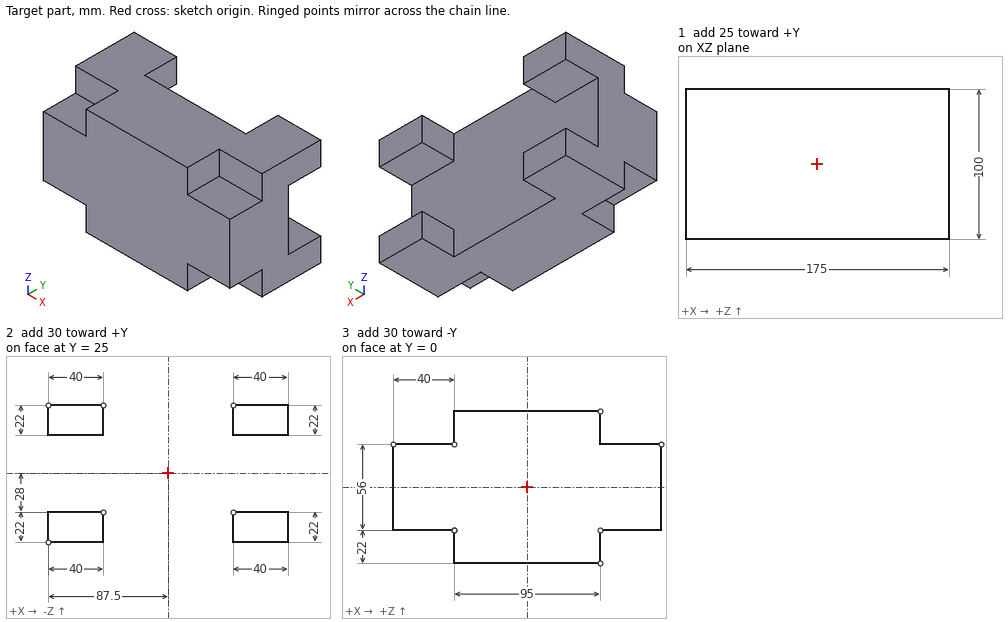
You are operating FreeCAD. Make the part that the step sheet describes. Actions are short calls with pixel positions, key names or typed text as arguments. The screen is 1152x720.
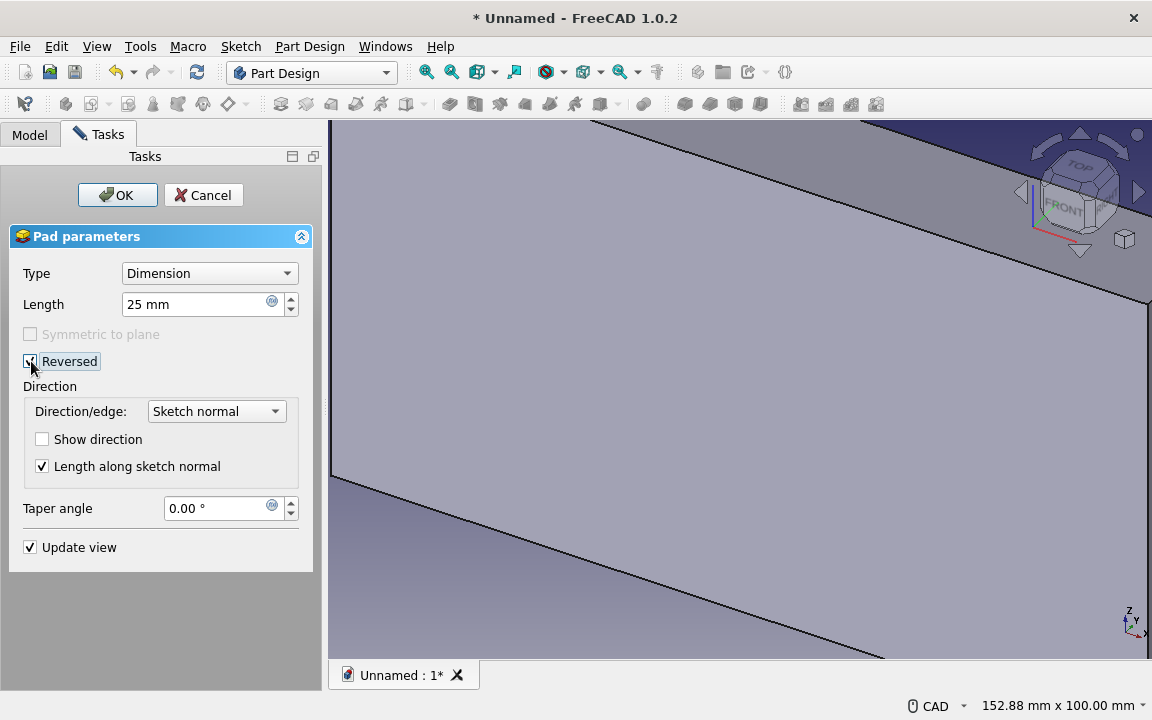
click(118, 195)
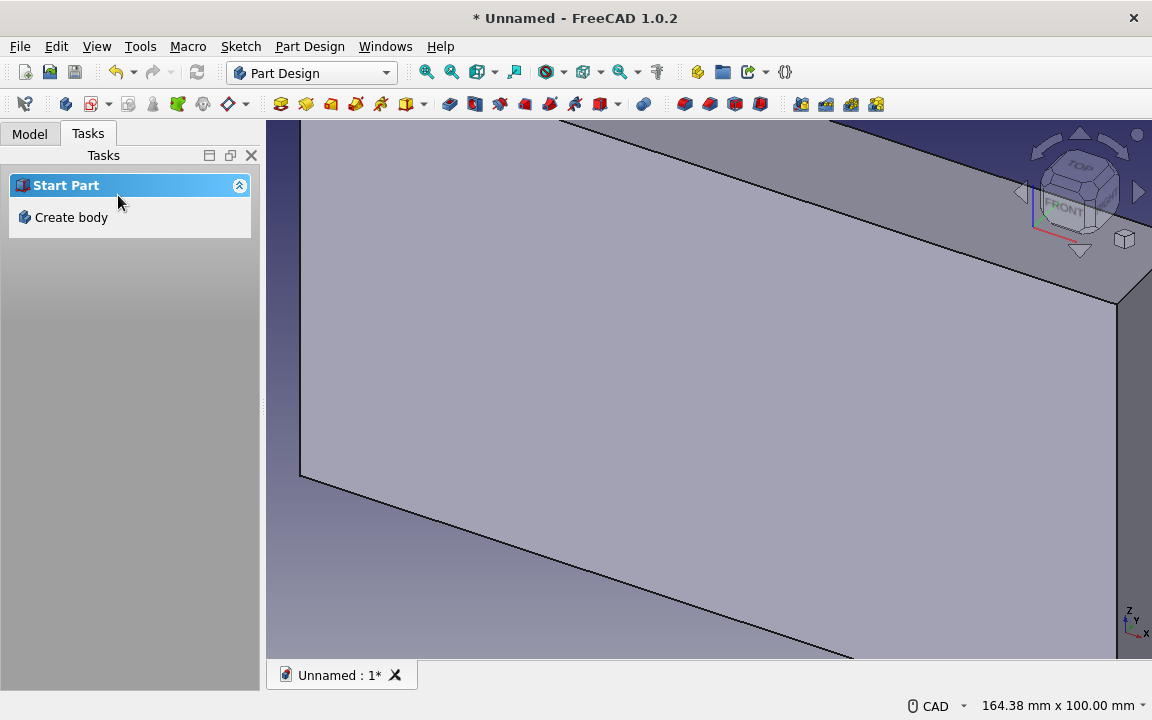
key(v)
key(f)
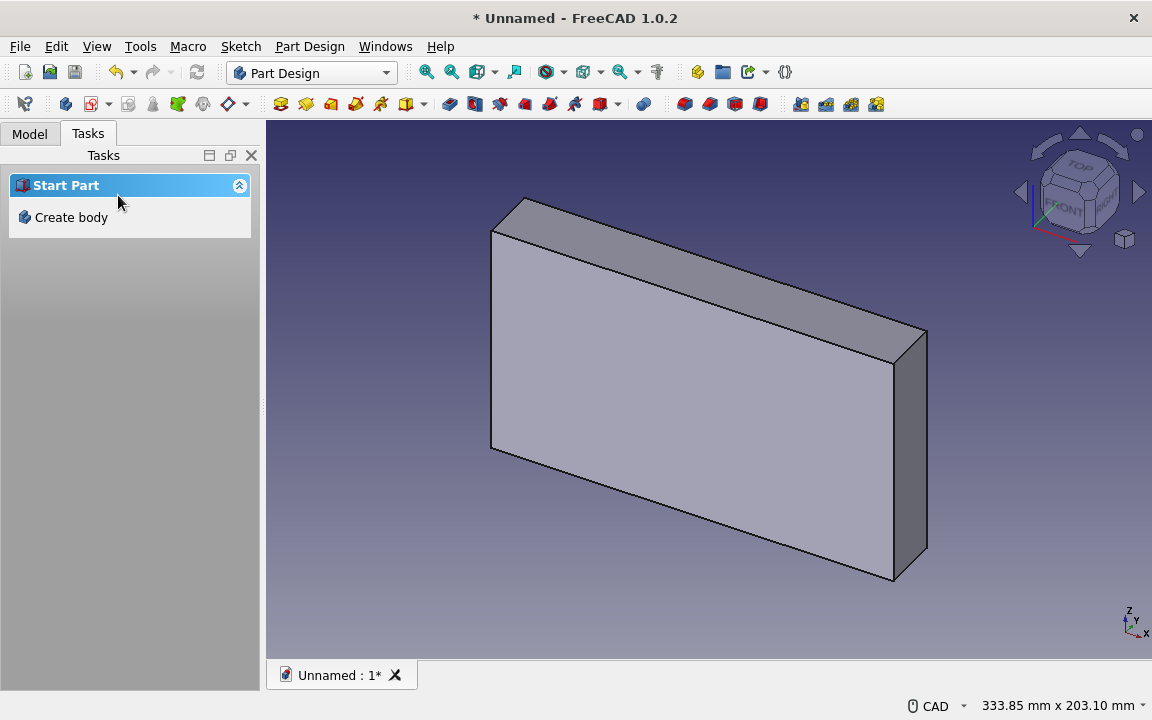
key(4)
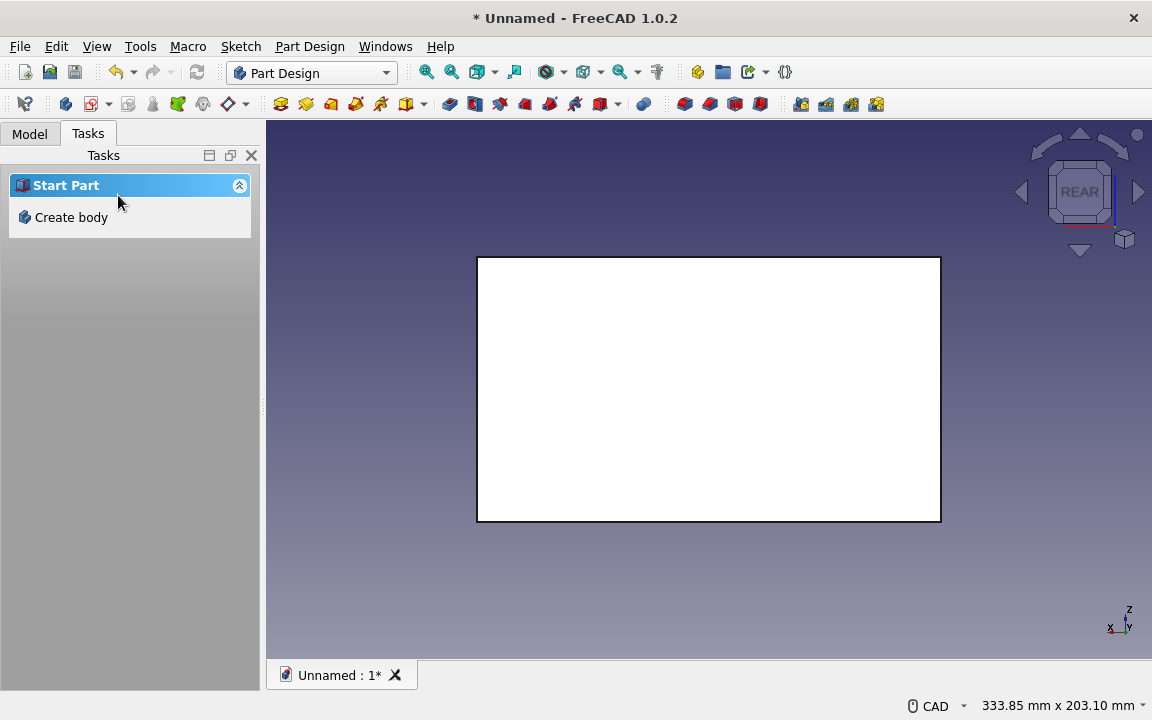
click(643, 389)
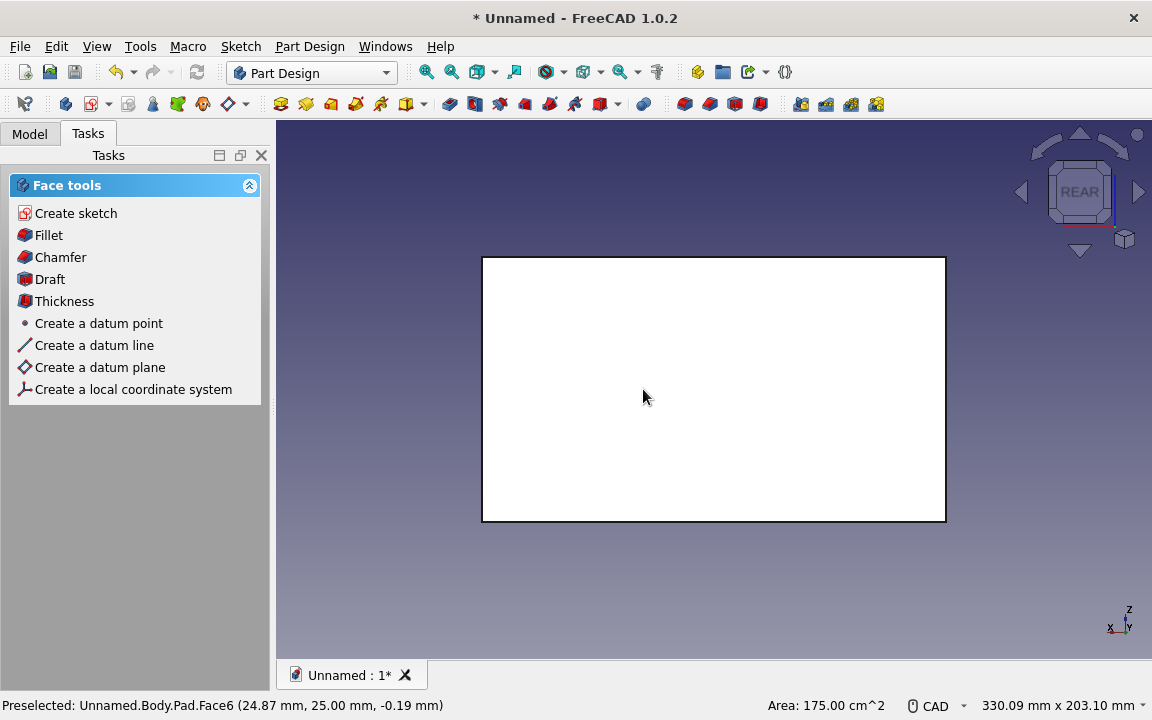
click(90, 104)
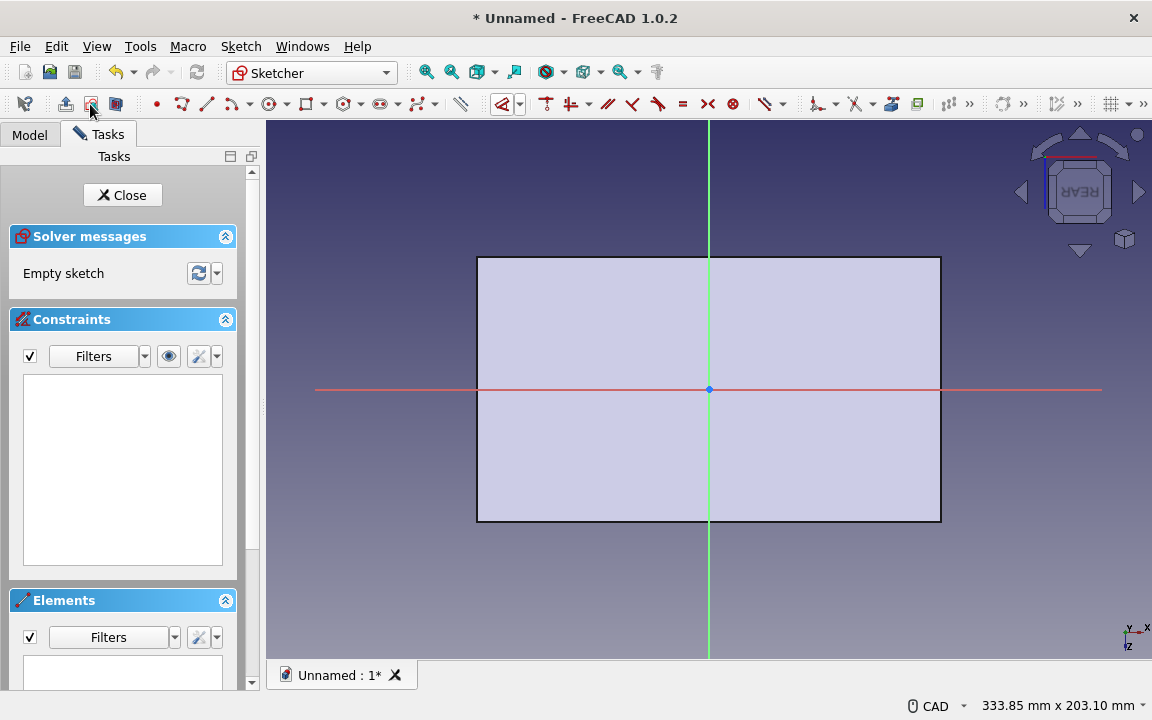
click(306, 104)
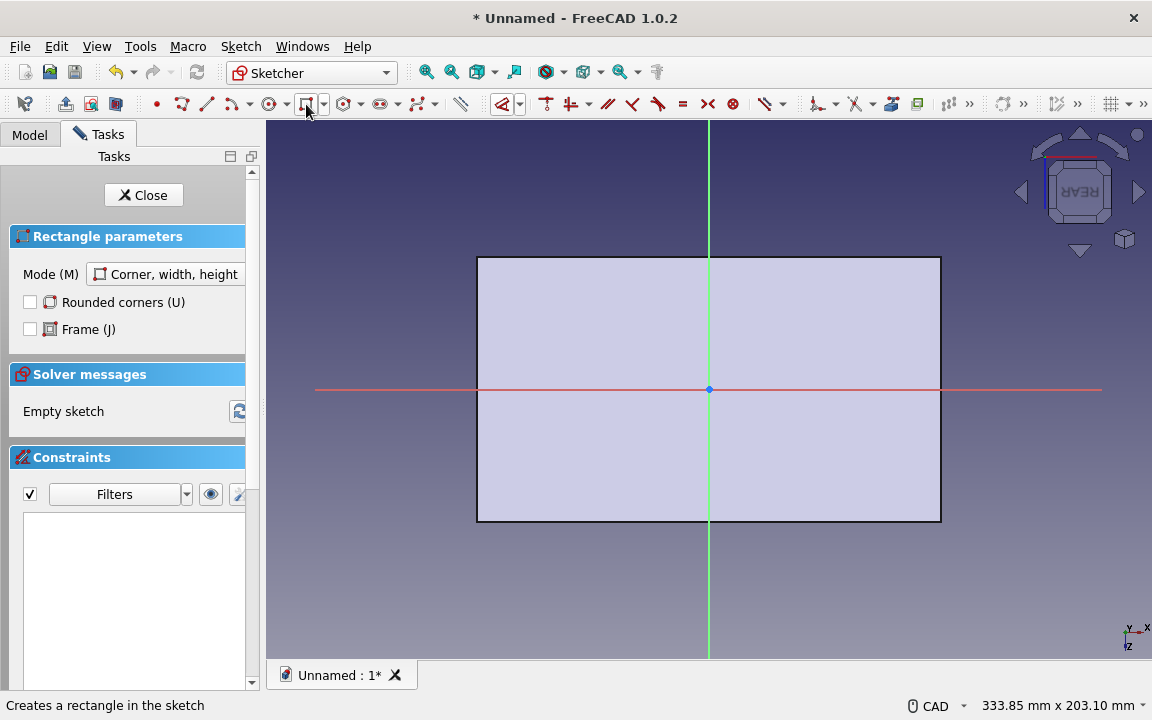
click(477, 464)
move(583, 522)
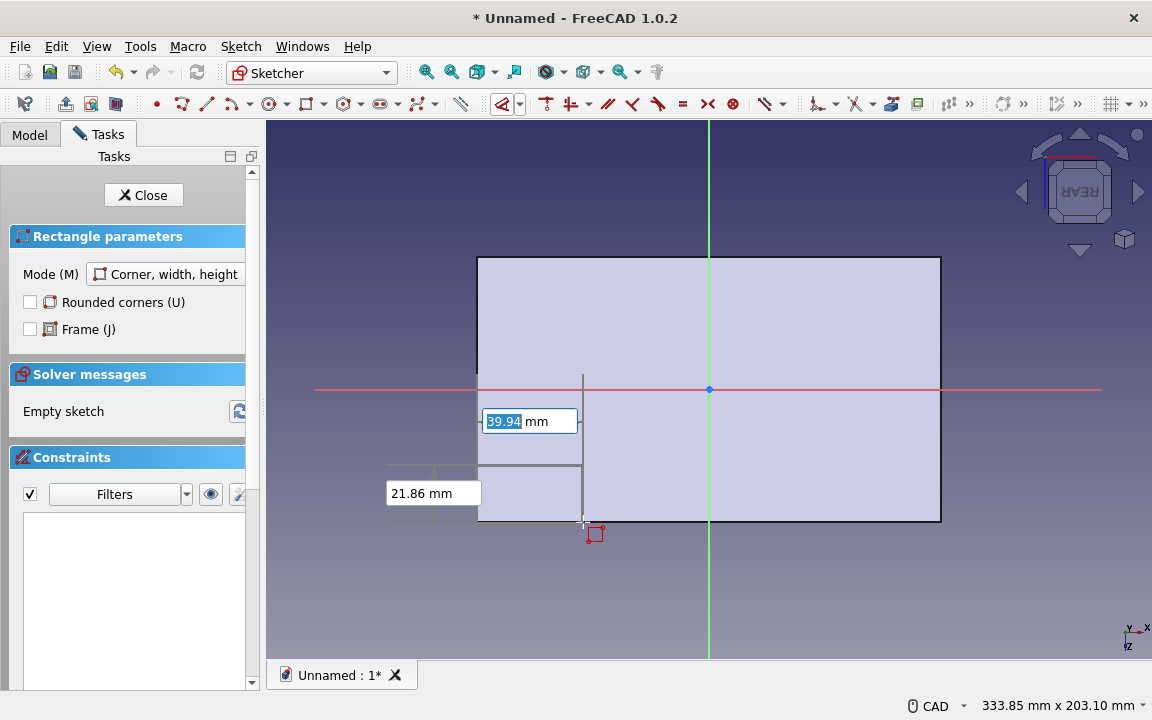
text(40)
key(Tab)
text(22)
key(Return)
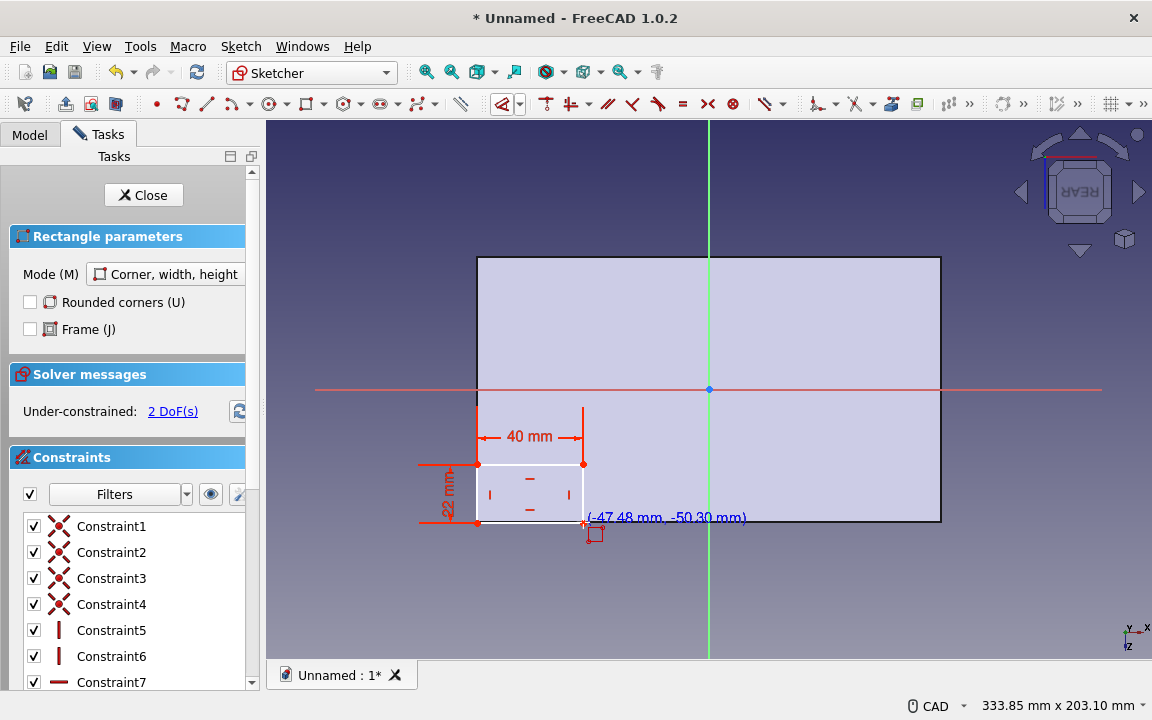
click(477, 257)
move(583, 315)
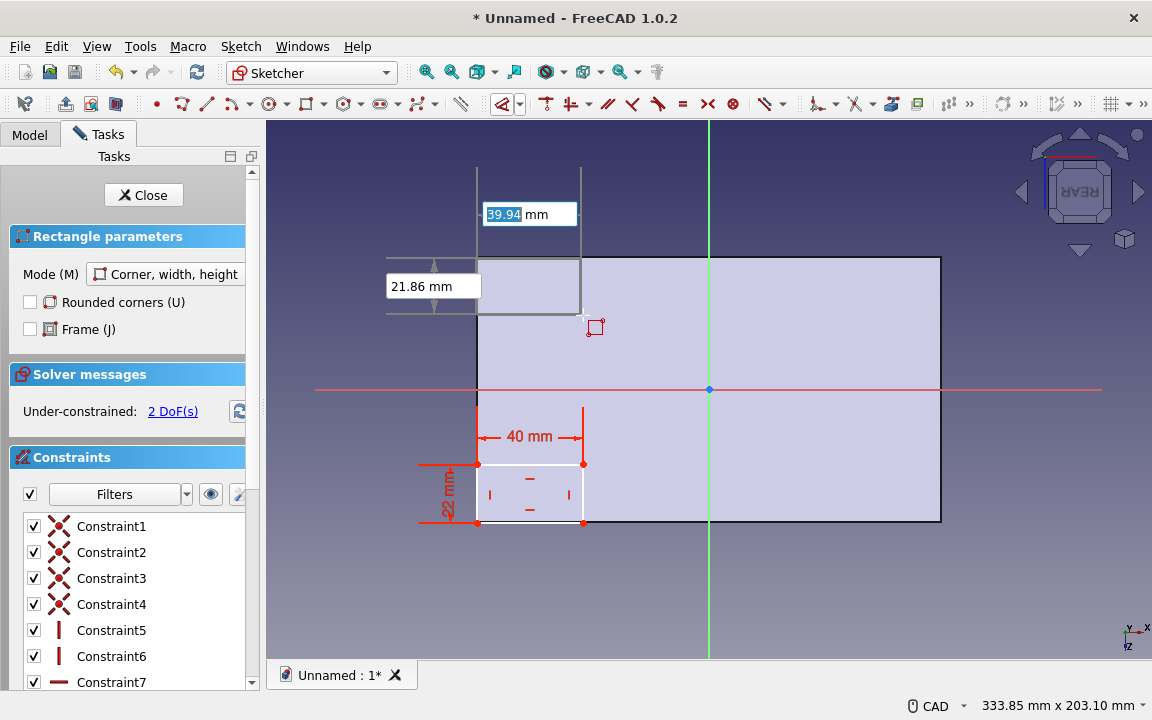
text(40)
key(Tab)
text(22)
key(Return)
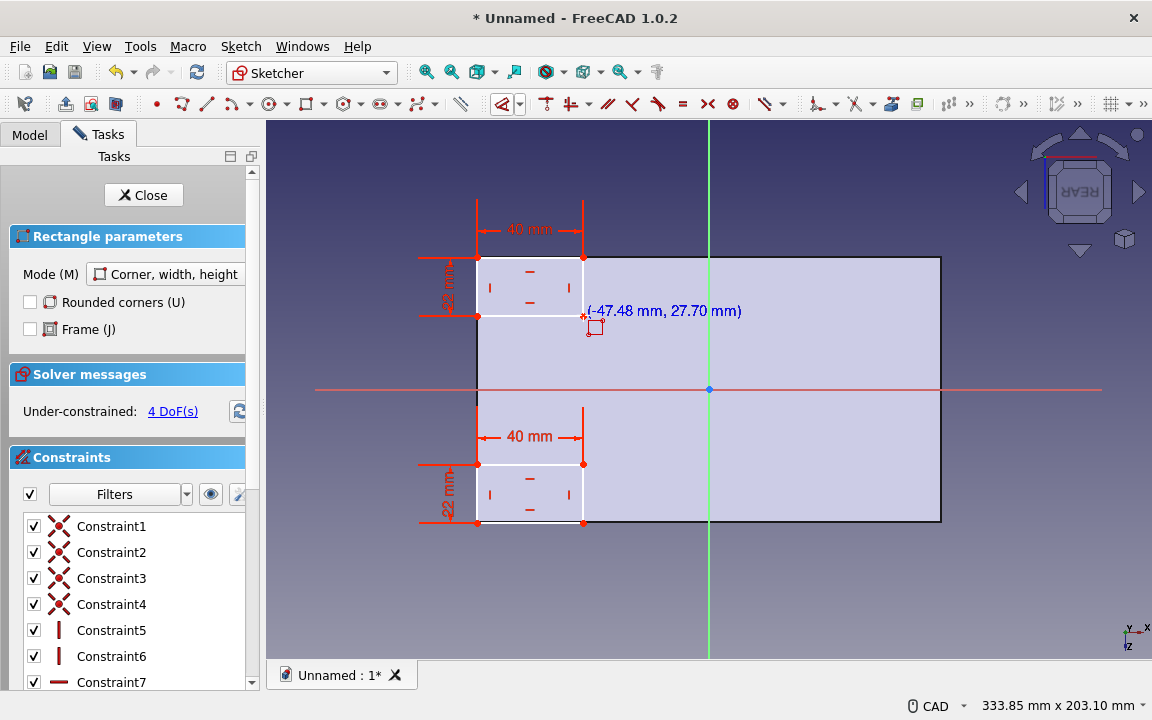
click(835, 257)
move(941, 315)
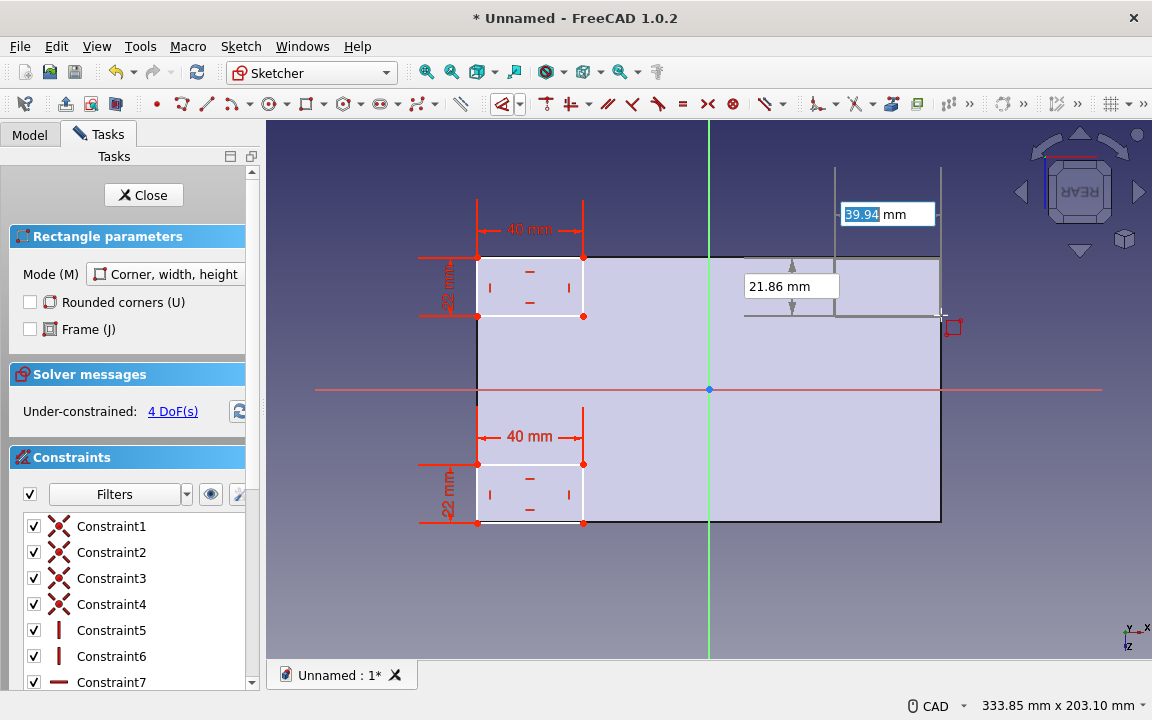
text(40)
key(Tab)
text(22)
key(Return)